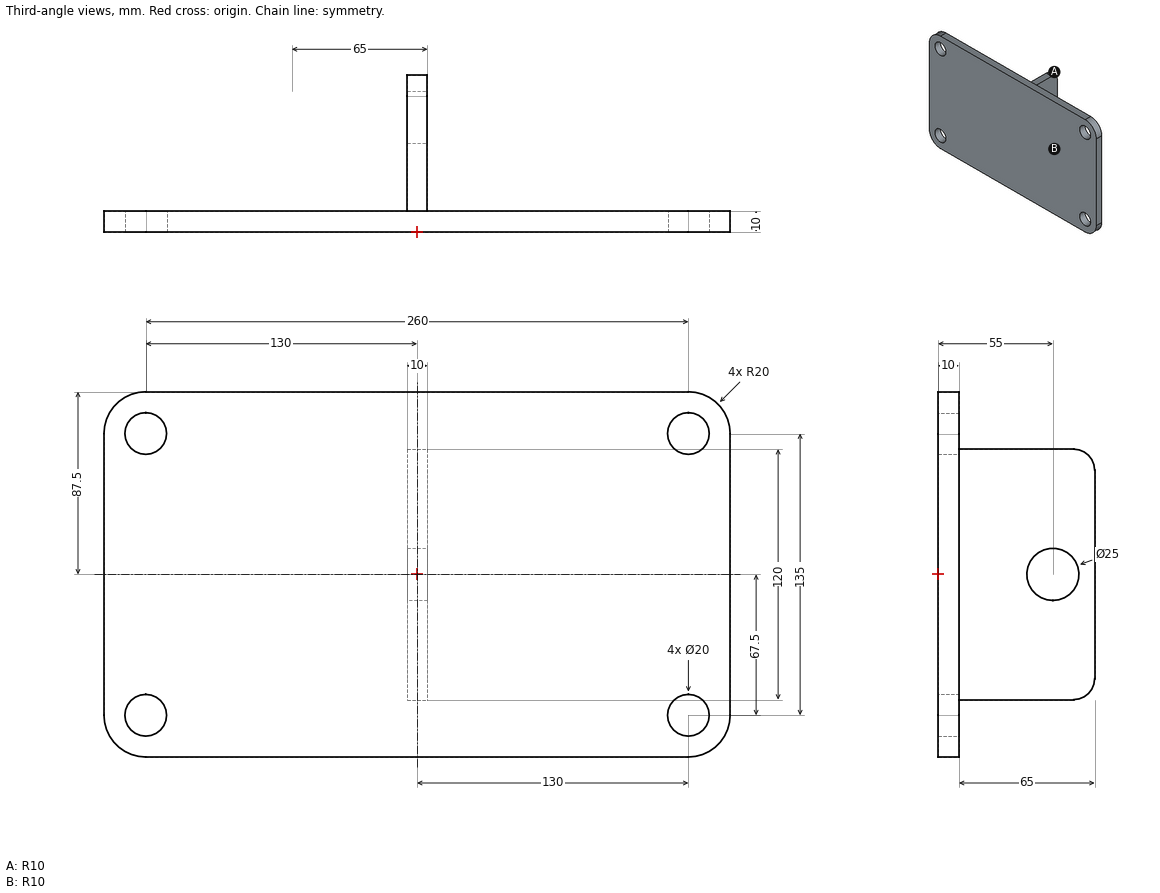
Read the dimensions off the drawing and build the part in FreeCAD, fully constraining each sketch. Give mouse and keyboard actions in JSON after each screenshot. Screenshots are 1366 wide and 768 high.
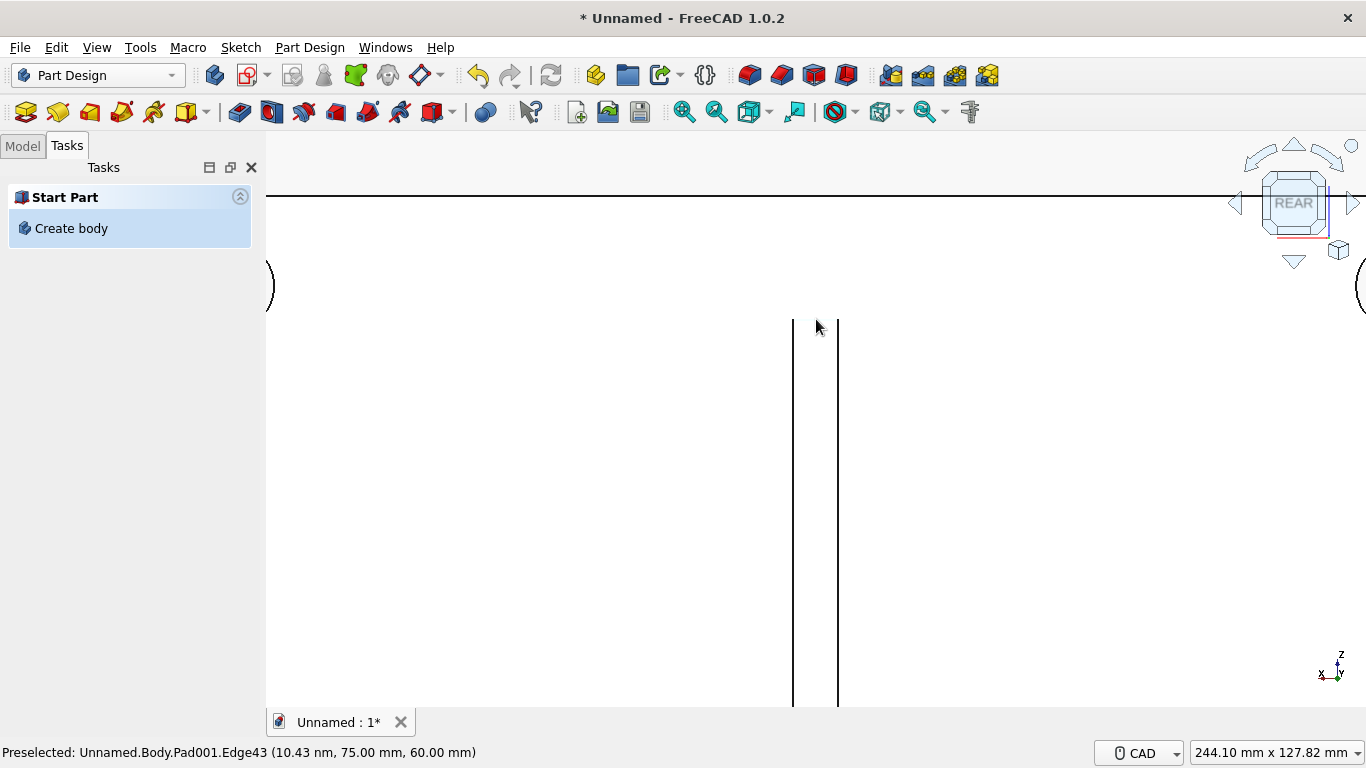
{"action": "left_click", "coordinate": [686, 112]}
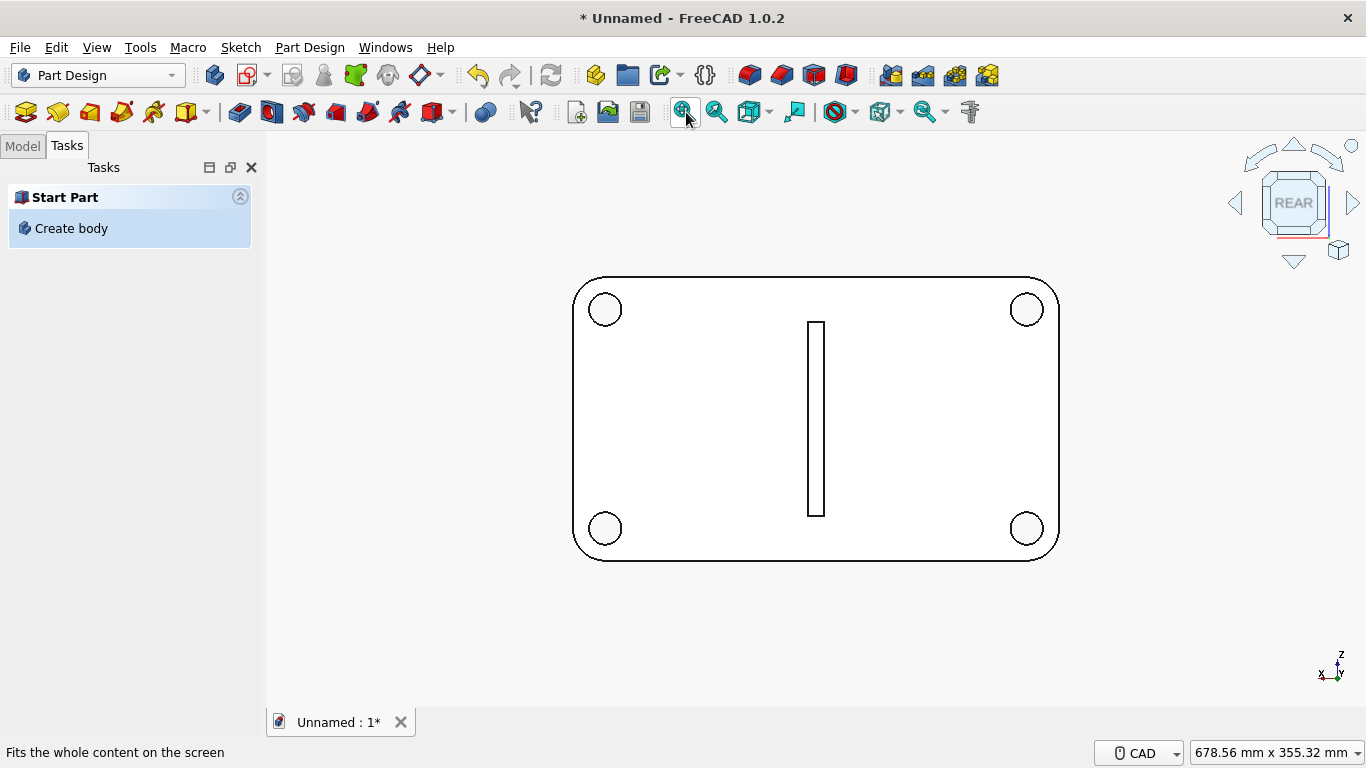
{"action": "key", "text": "0"}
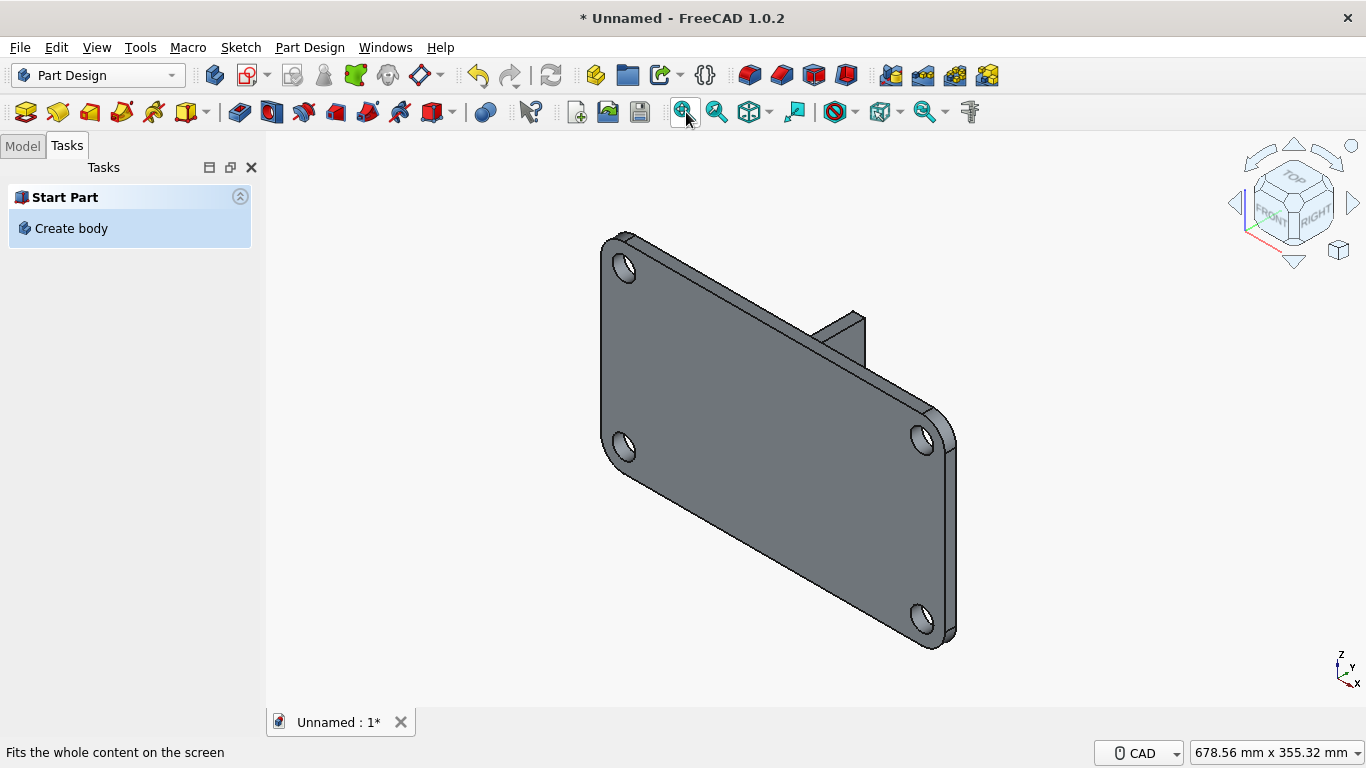
{"action": "scroll", "coordinate": [859, 314], "scroll_direction": "up", "scroll_amount": 5}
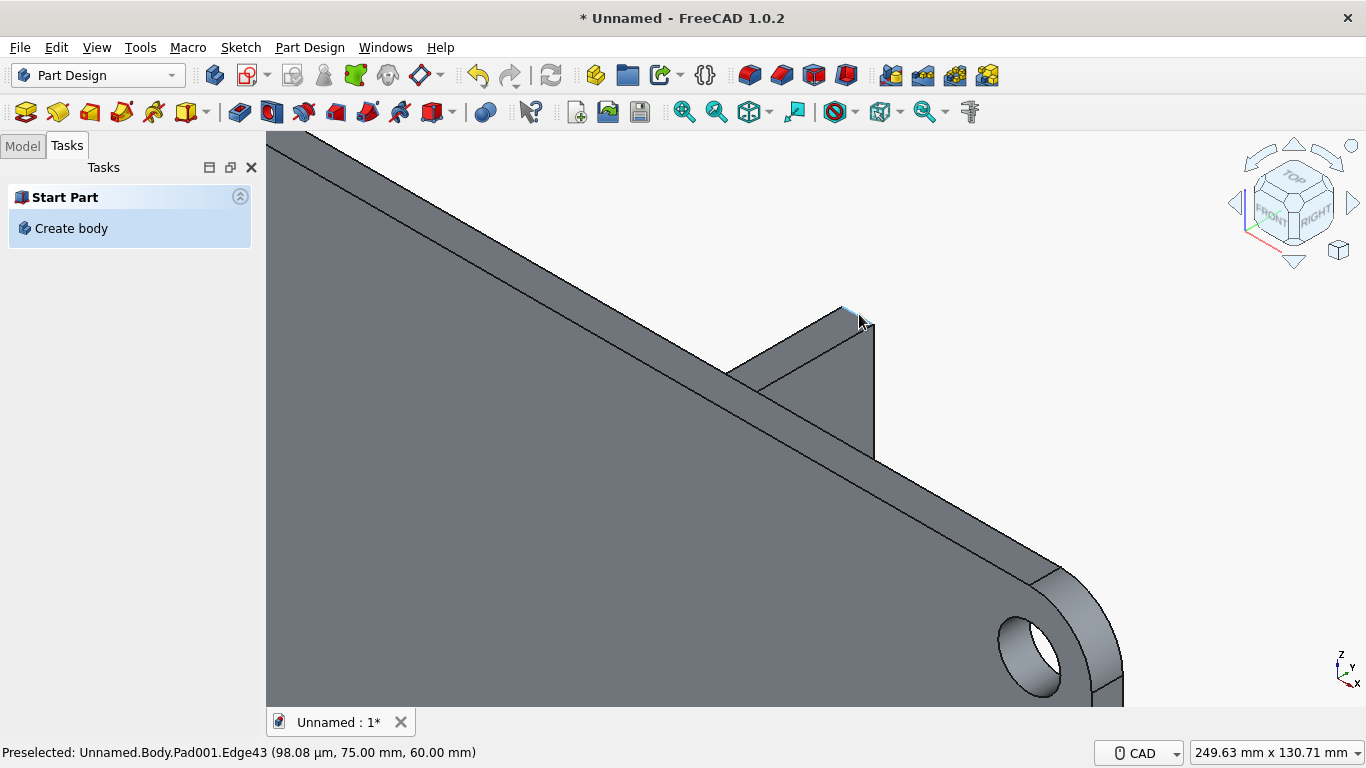
{"action": "left_click", "coordinate": [686, 112]}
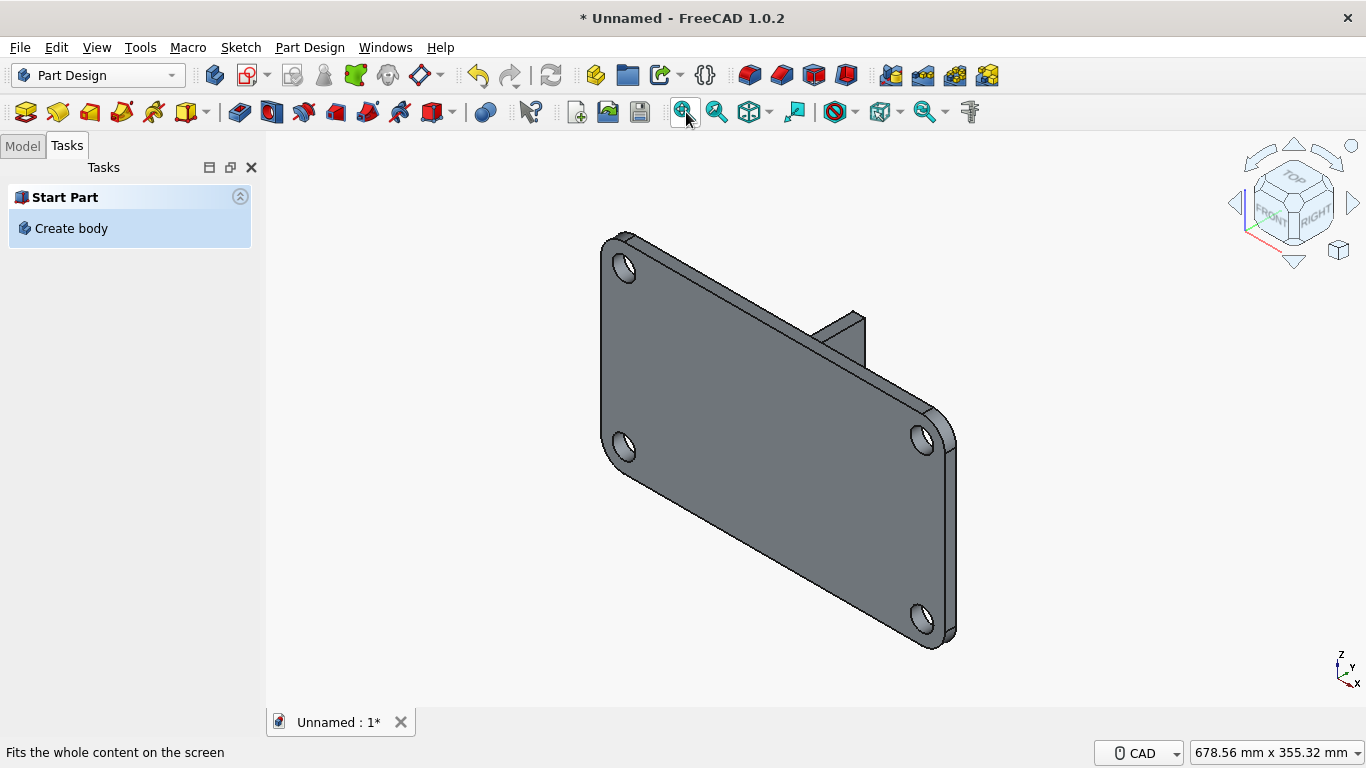
{"action": "key", "text": "2"}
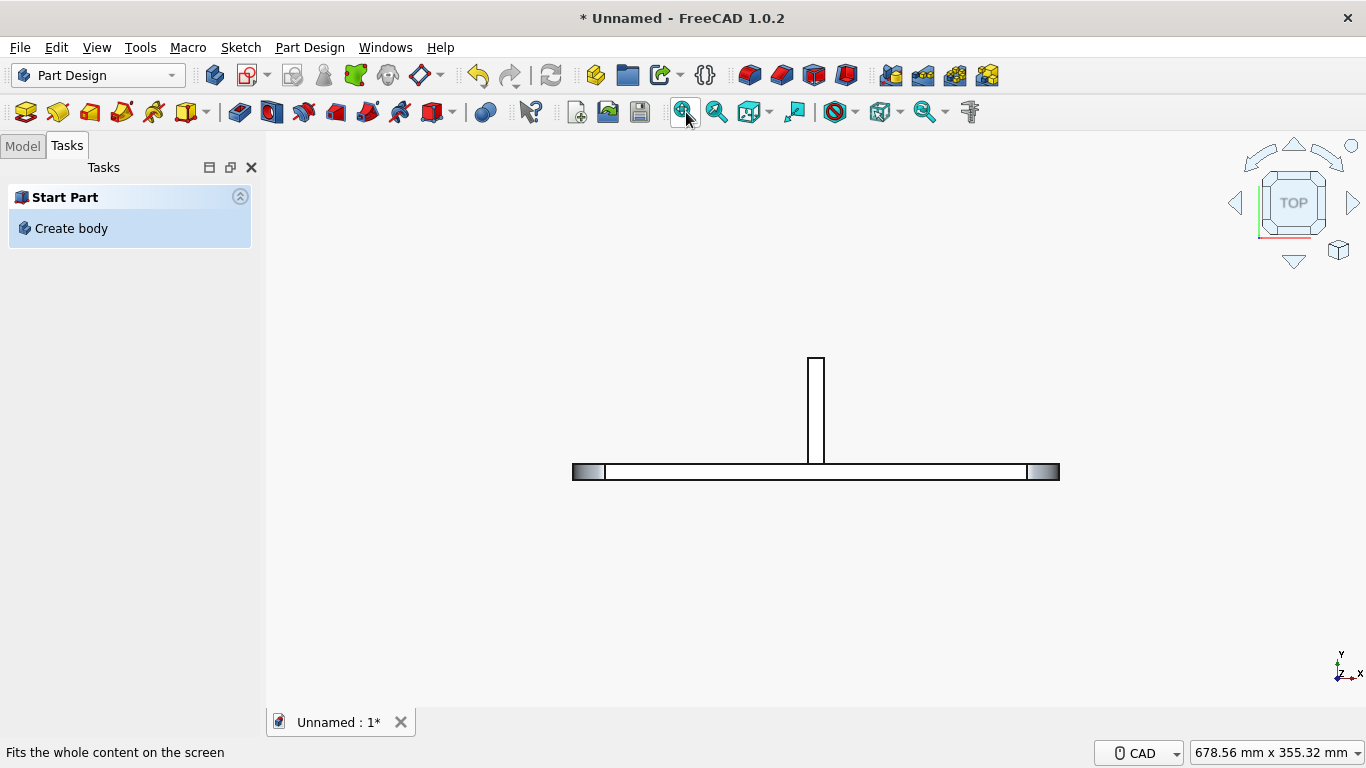
{"action": "left_click", "coordinate": [686, 112]}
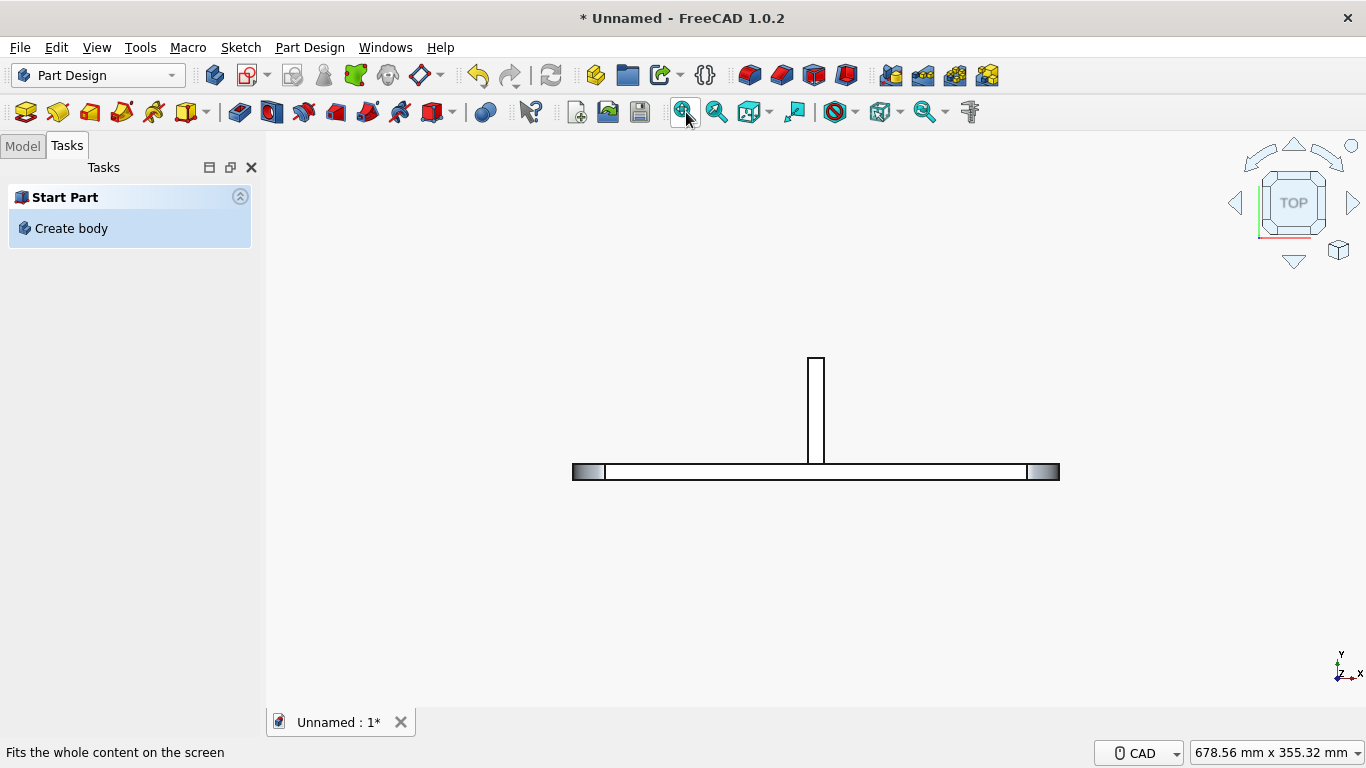
{"action": "left_click", "coordinate": [816, 357]}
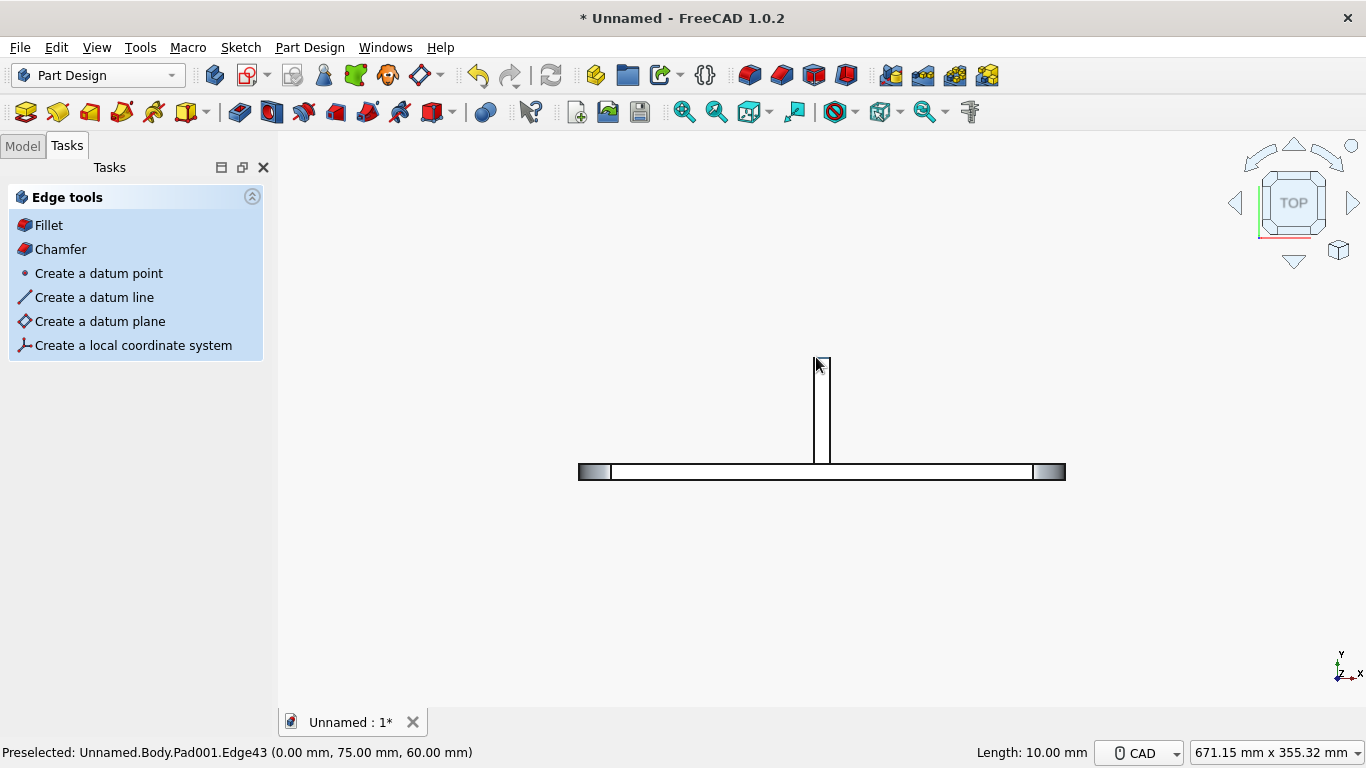
{"action": "left_click", "coordinate": [750, 76]}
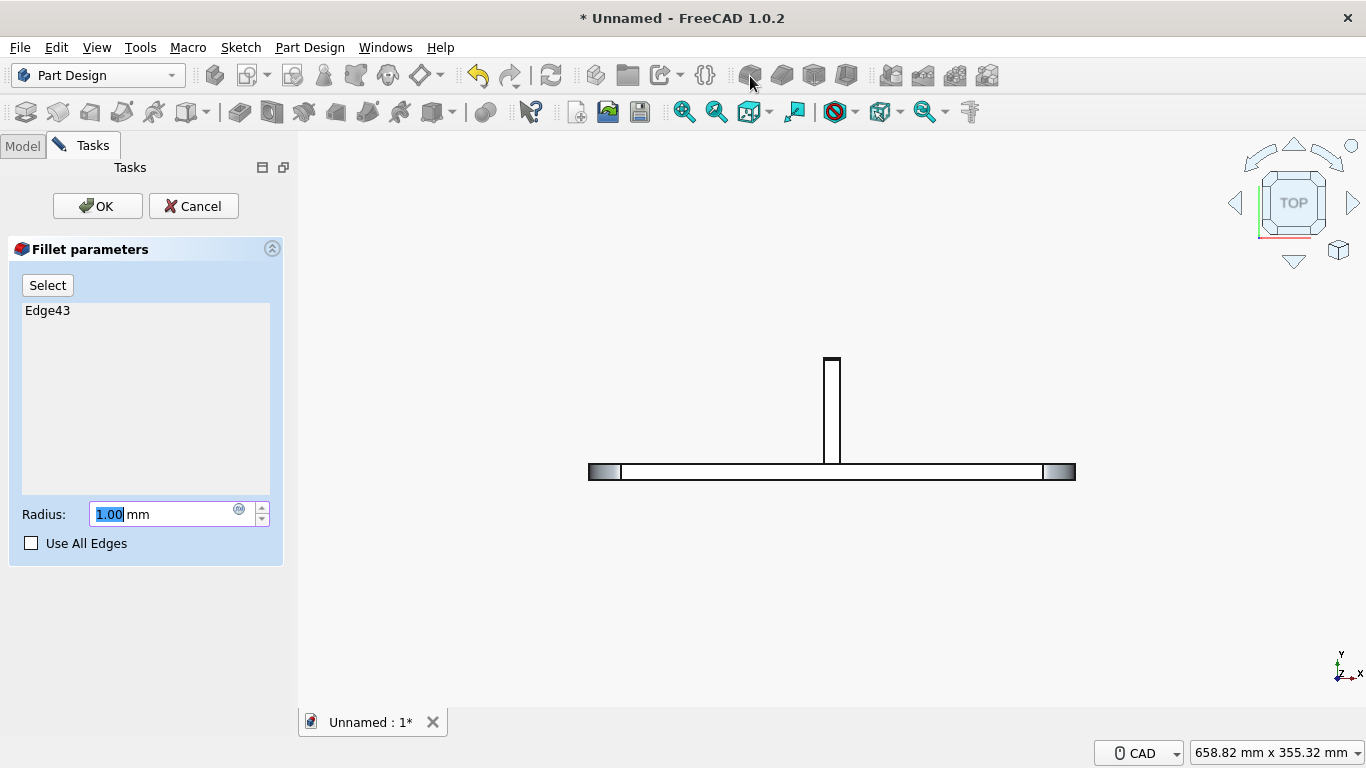
{"action": "type", "text": "10"}
{"action": "key", "text": "Tab"}